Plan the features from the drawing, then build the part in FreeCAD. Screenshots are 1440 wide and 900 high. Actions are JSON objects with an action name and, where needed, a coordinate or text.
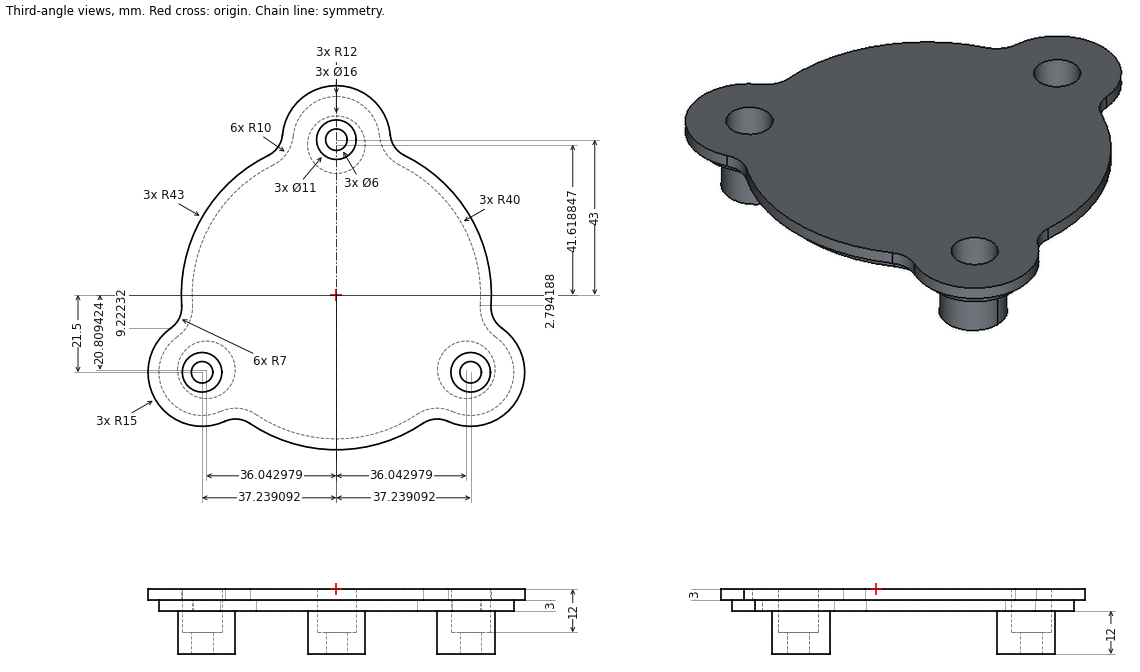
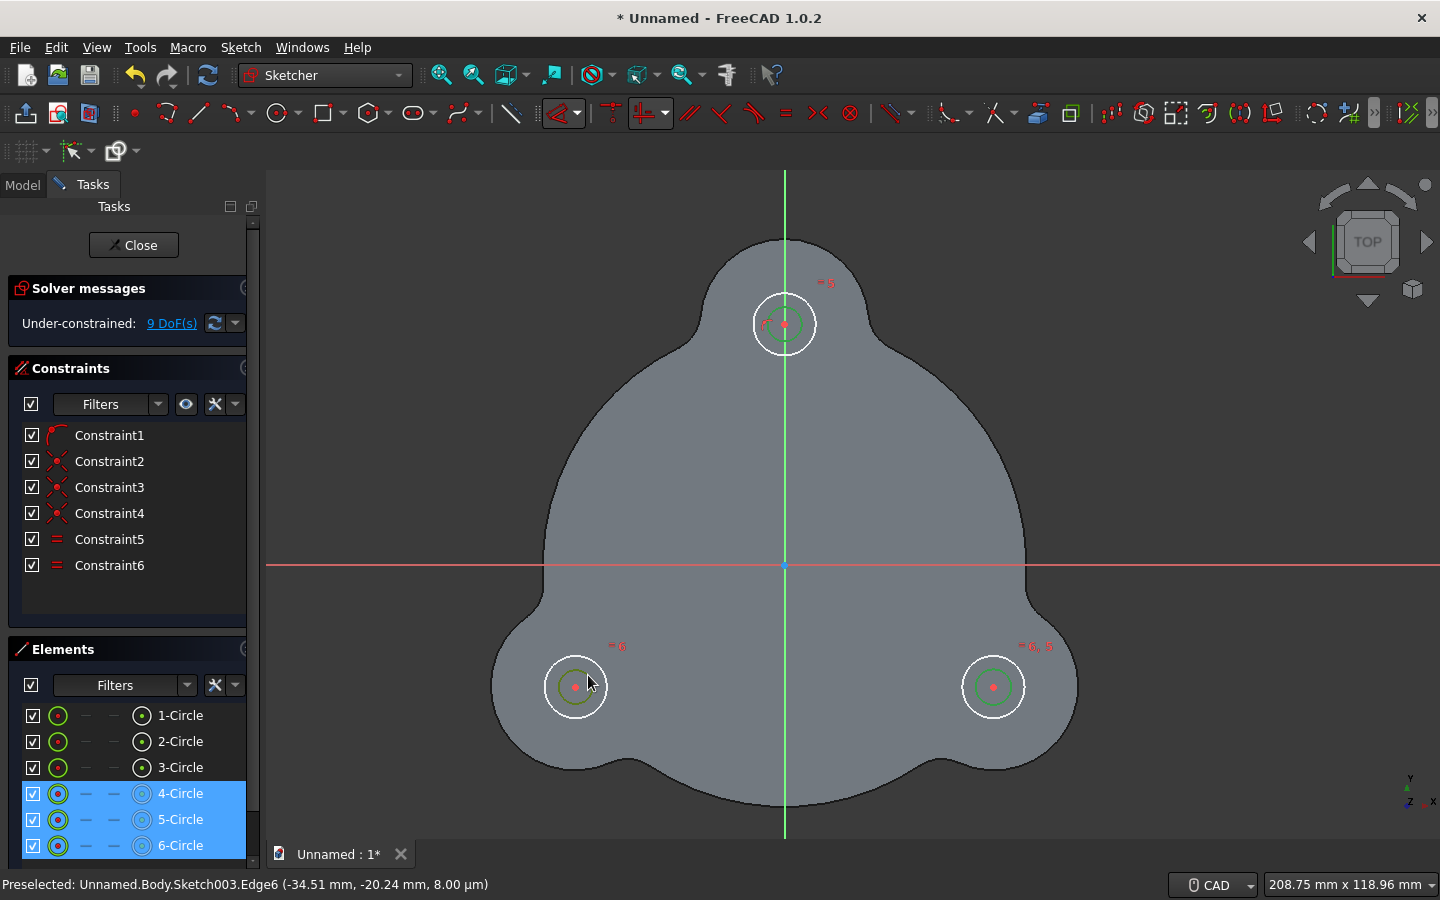
{"action": "left_click", "coordinate": [786, 114]}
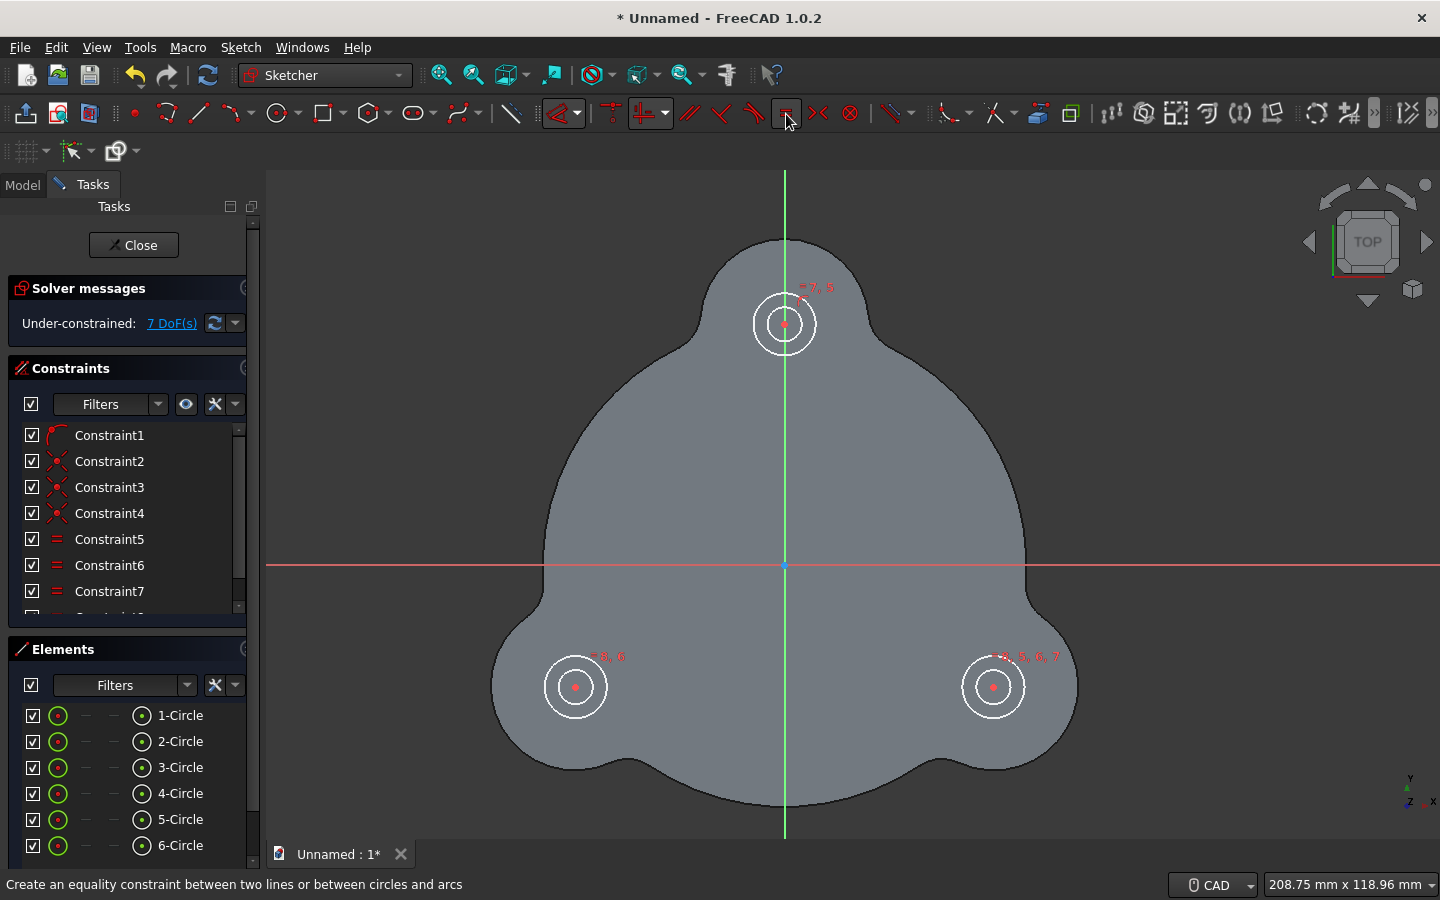
{"action": "left_click", "coordinate": [993, 687]}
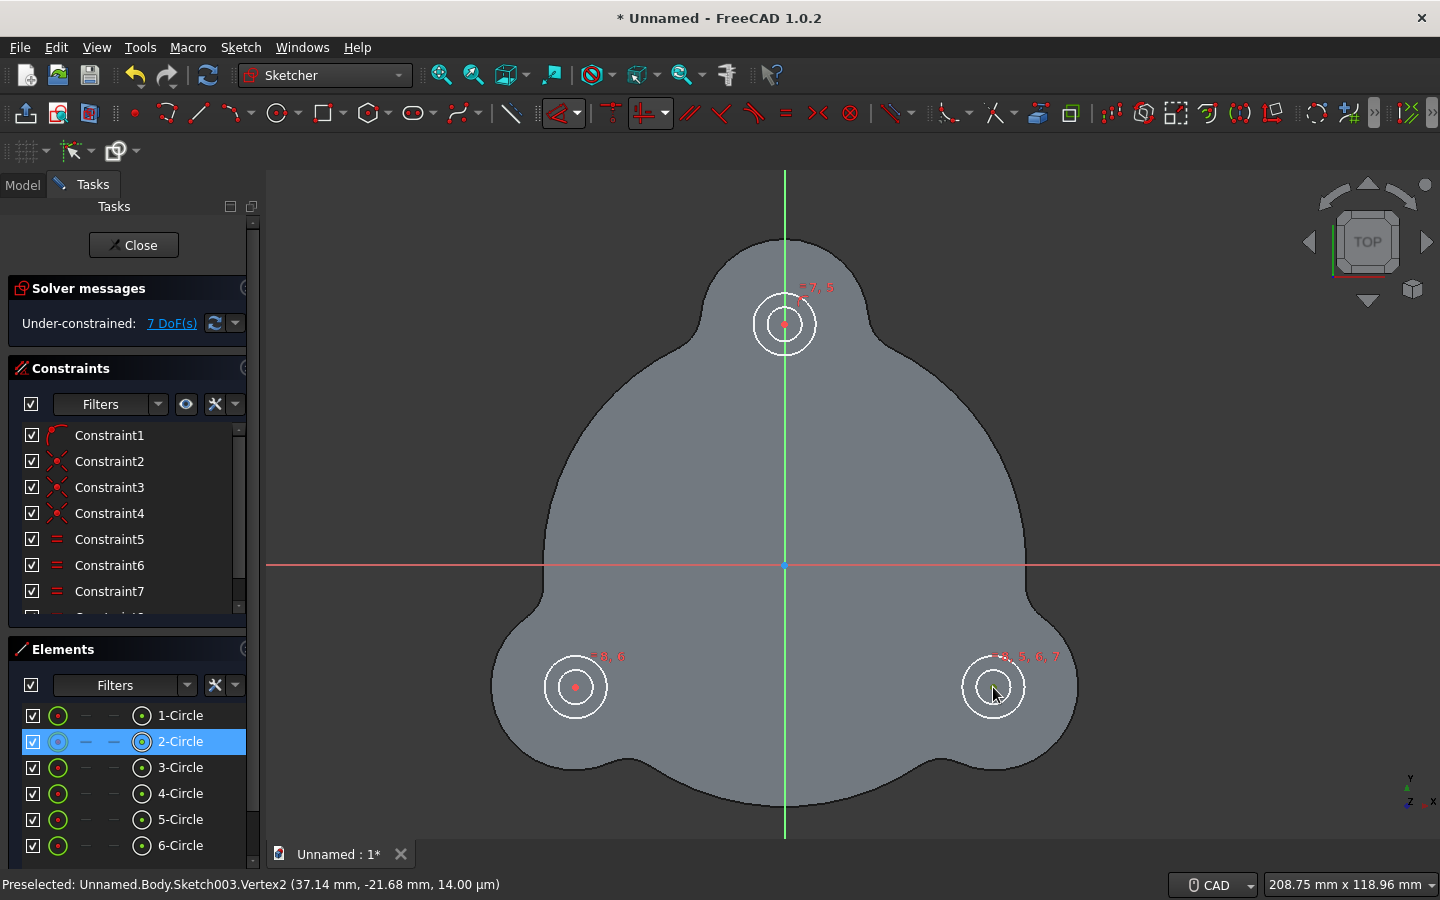
{"action": "left_click", "coordinate": [576, 687]}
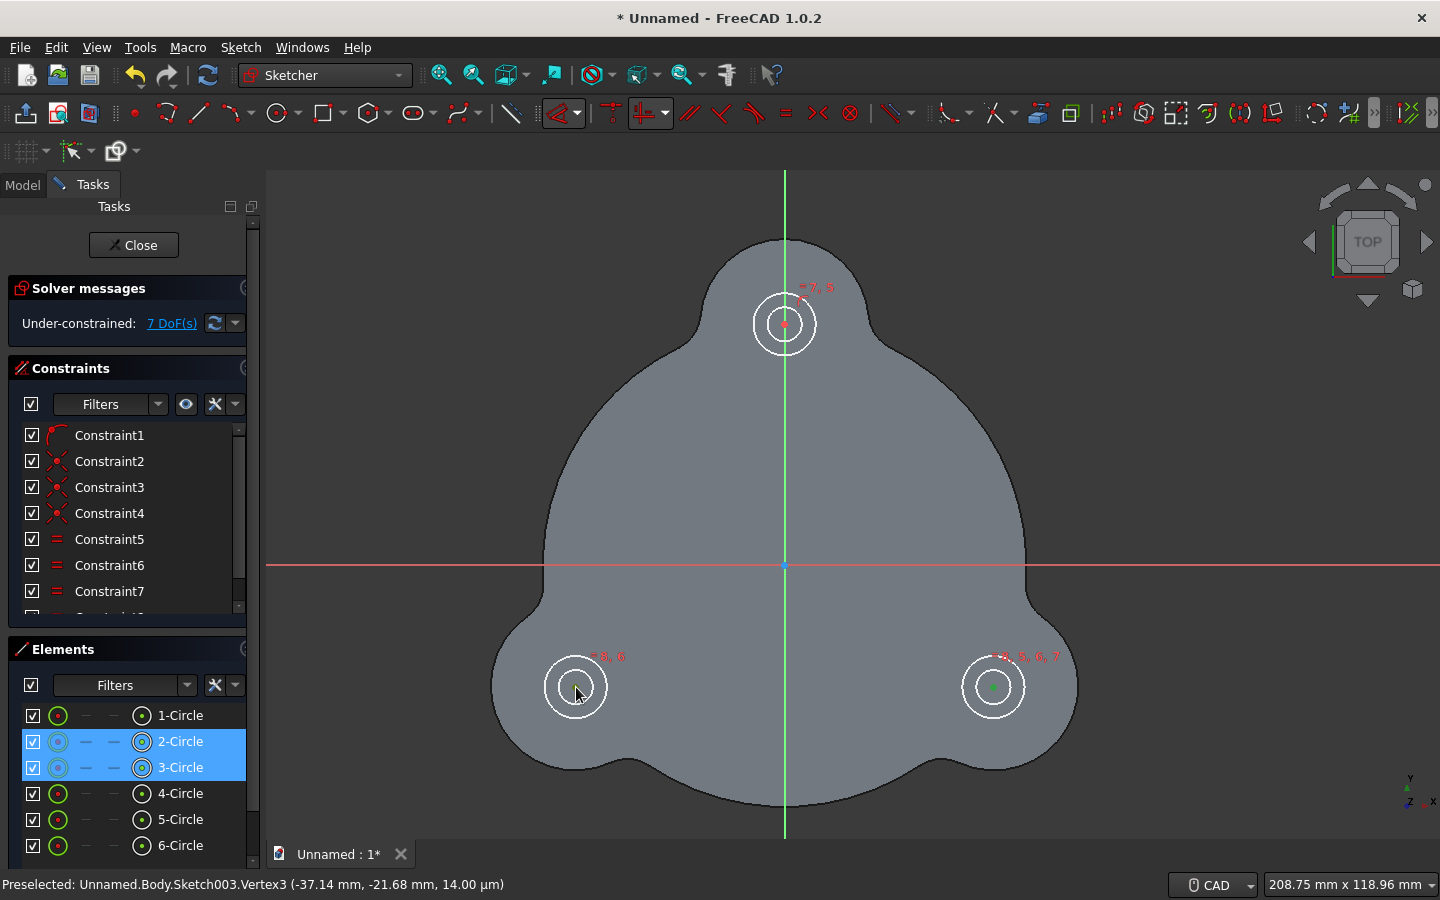
{"action": "left_click", "coordinate": [668, 114]}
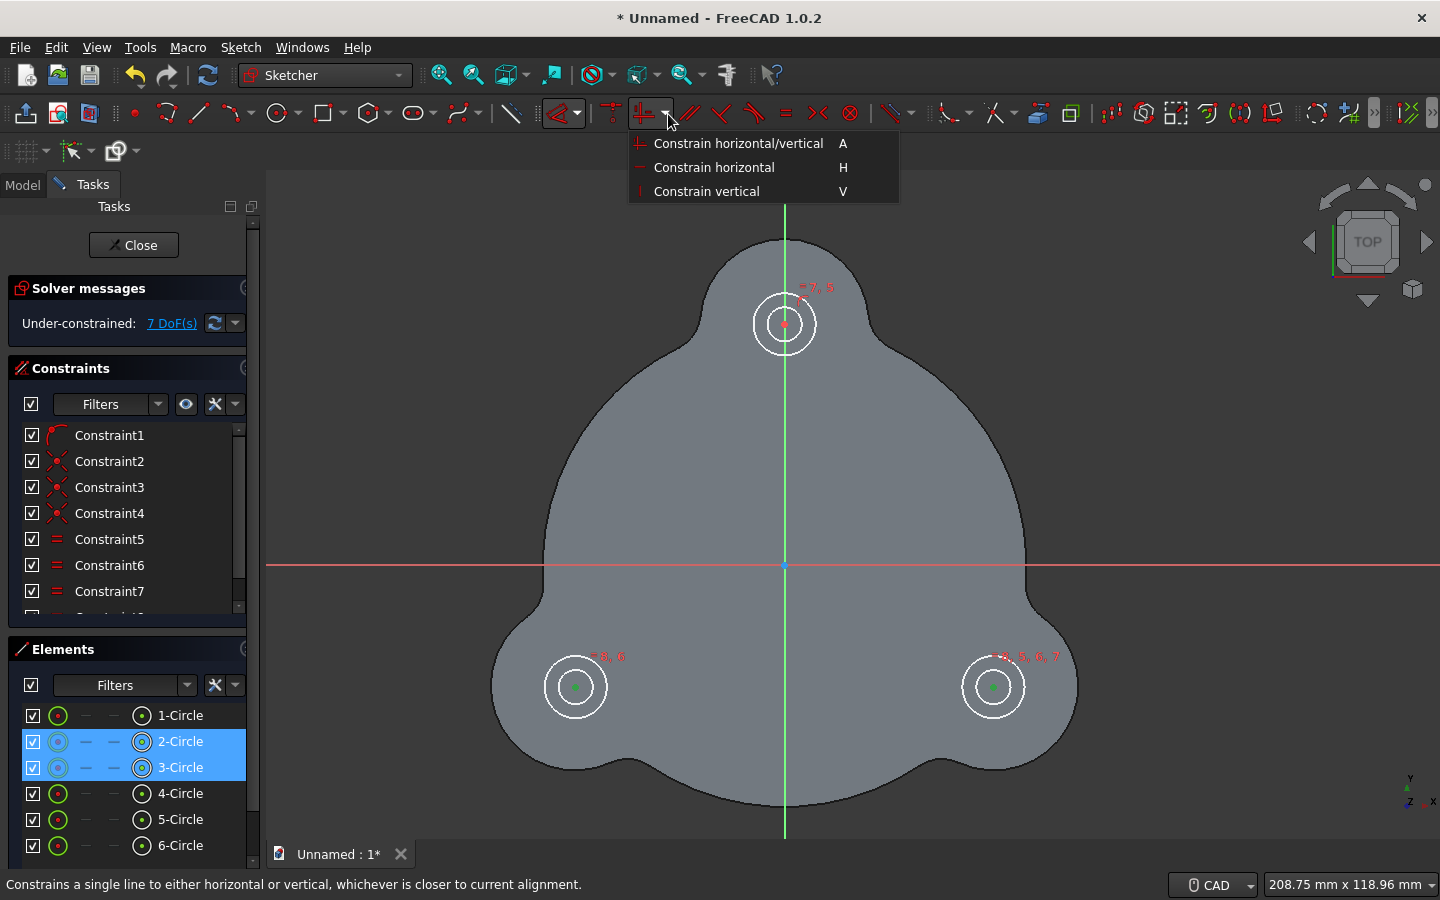
{"action": "left_click", "coordinate": [764, 167]}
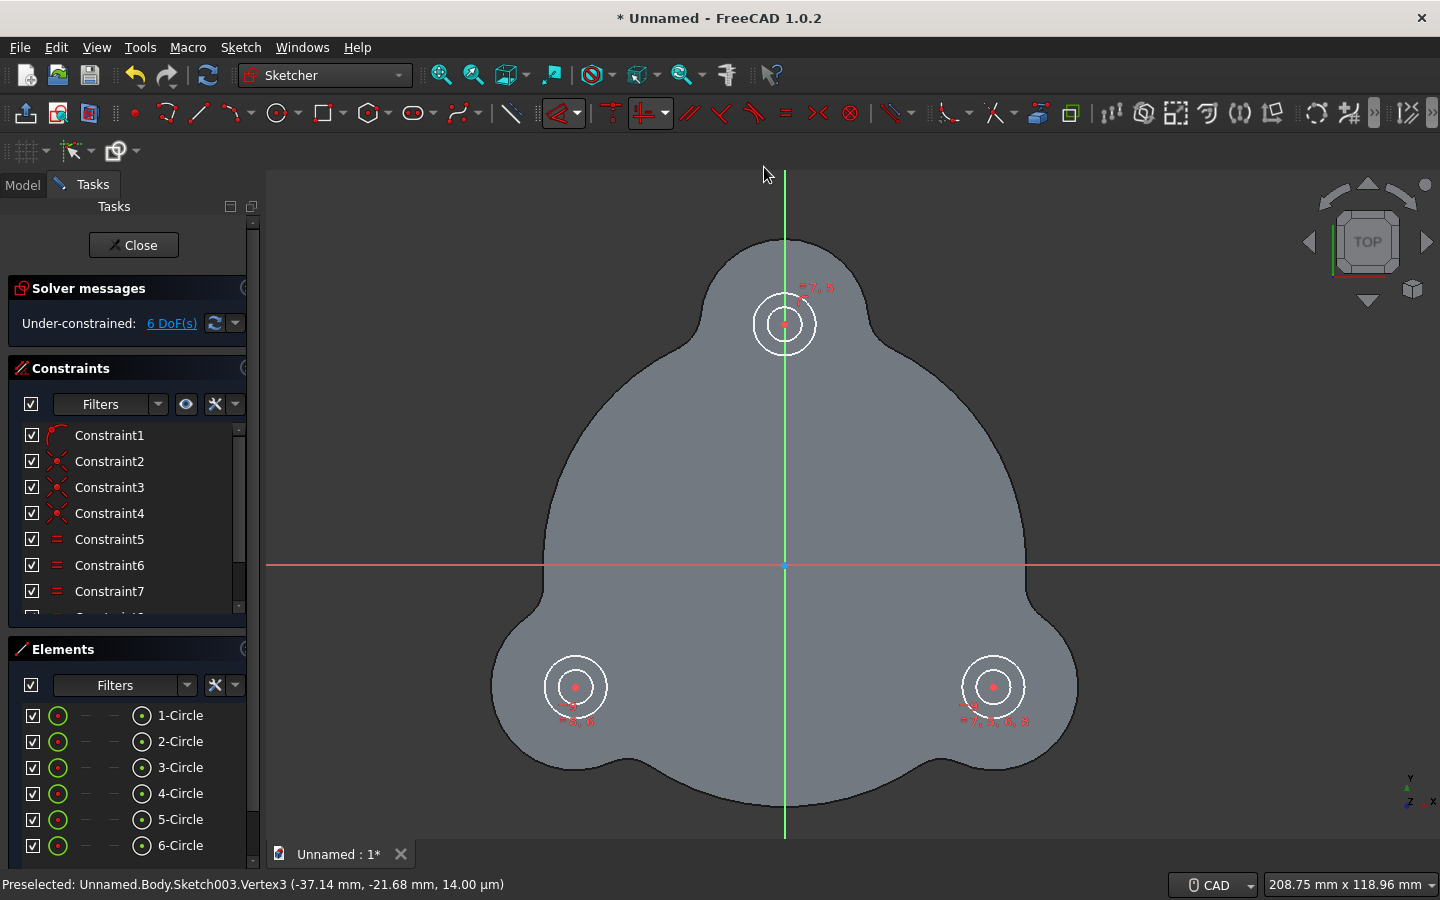
{"action": "left_click", "coordinate": [763, 302]}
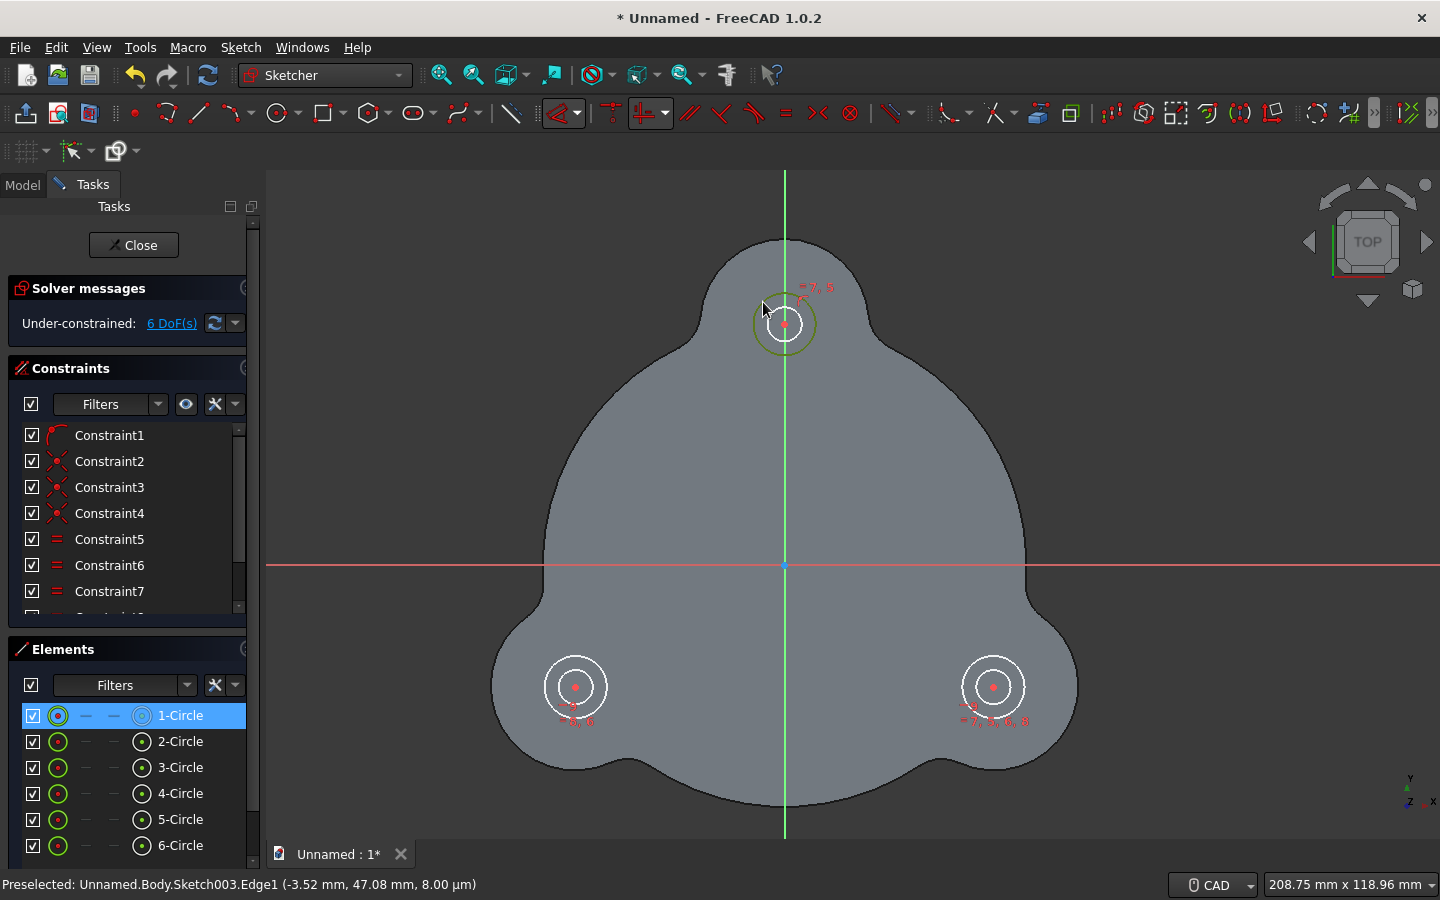
{"action": "left_click", "coordinate": [580, 114]}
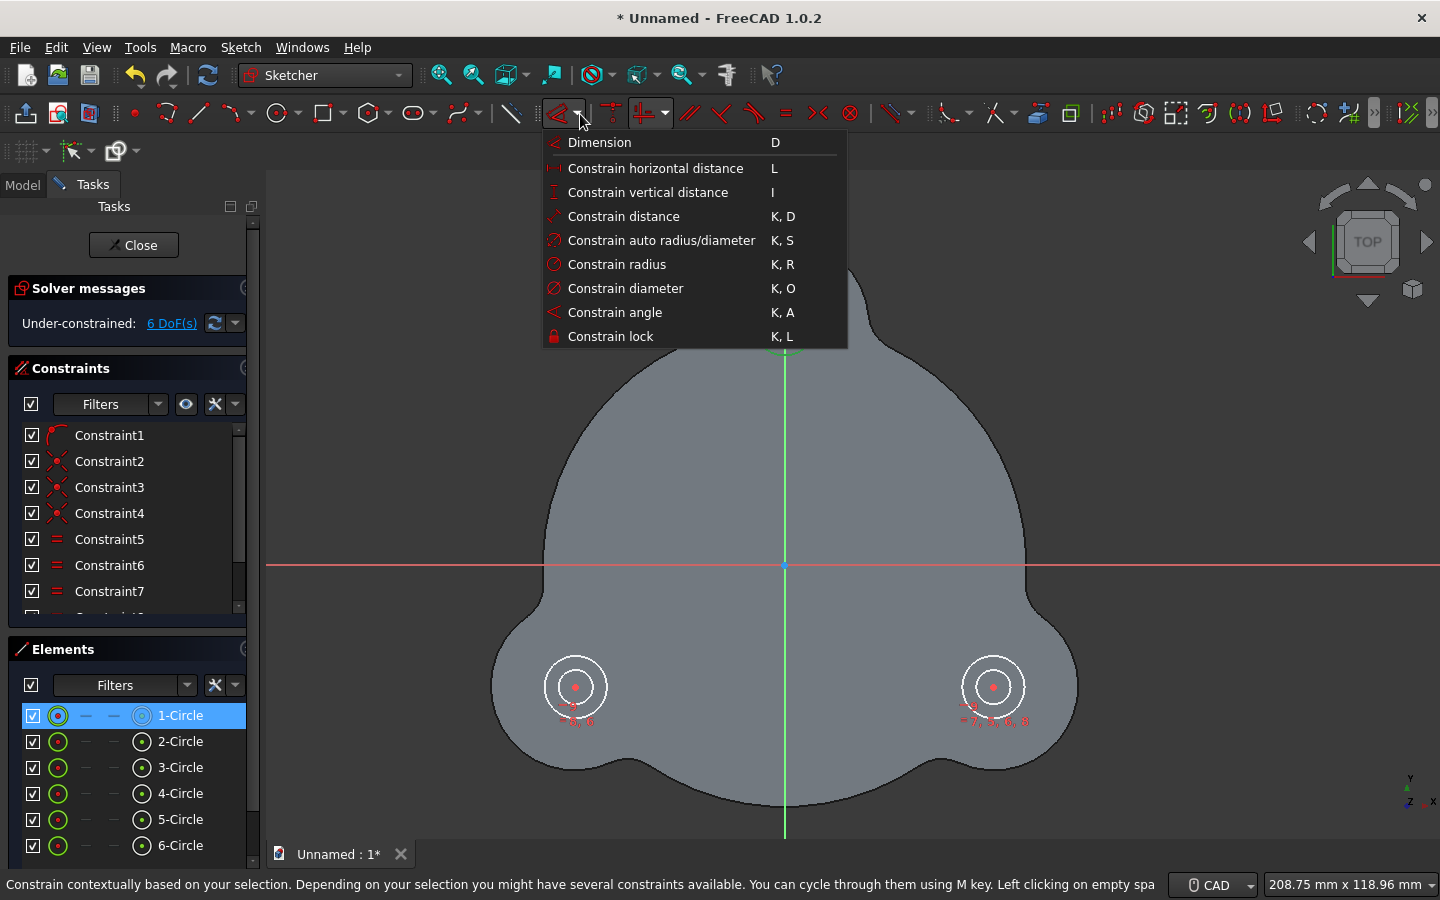
{"action": "left_click", "coordinate": [695, 288]}